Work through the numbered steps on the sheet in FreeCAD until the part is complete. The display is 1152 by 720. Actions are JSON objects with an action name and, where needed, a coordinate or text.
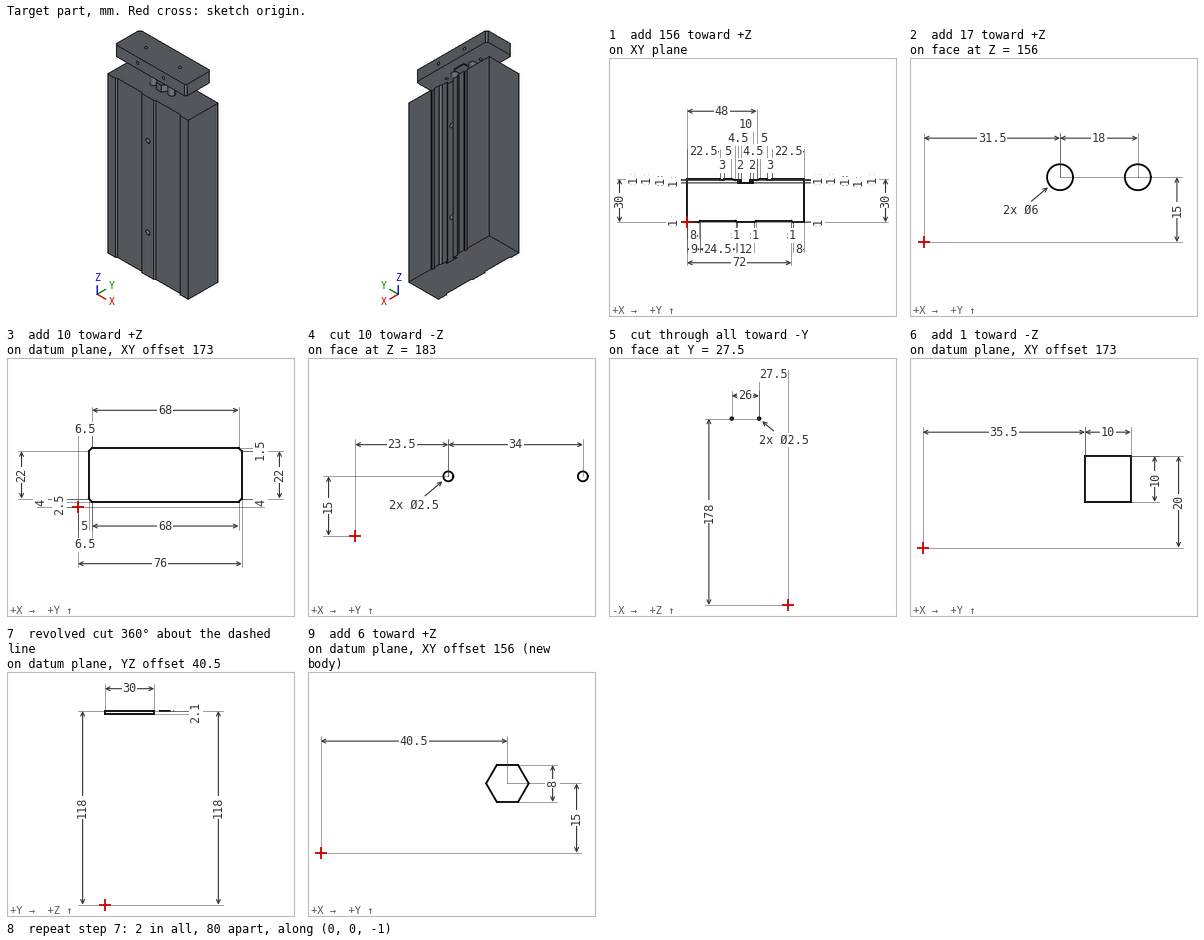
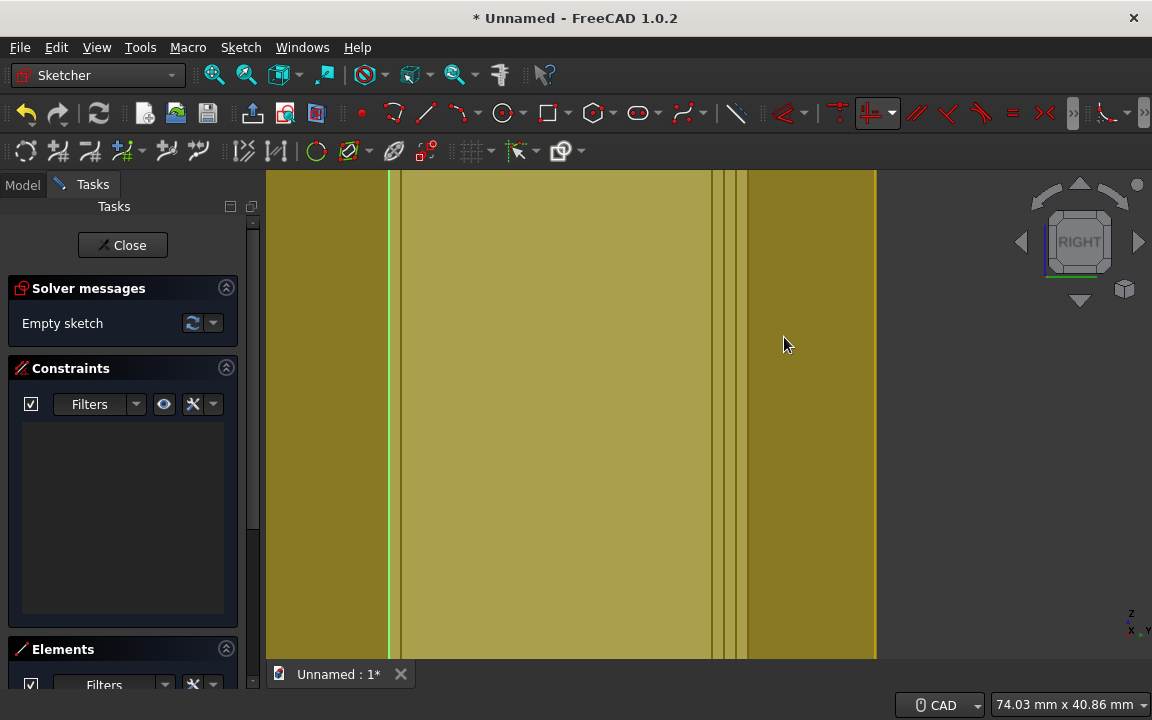
{"action": "key", "text": "g r"}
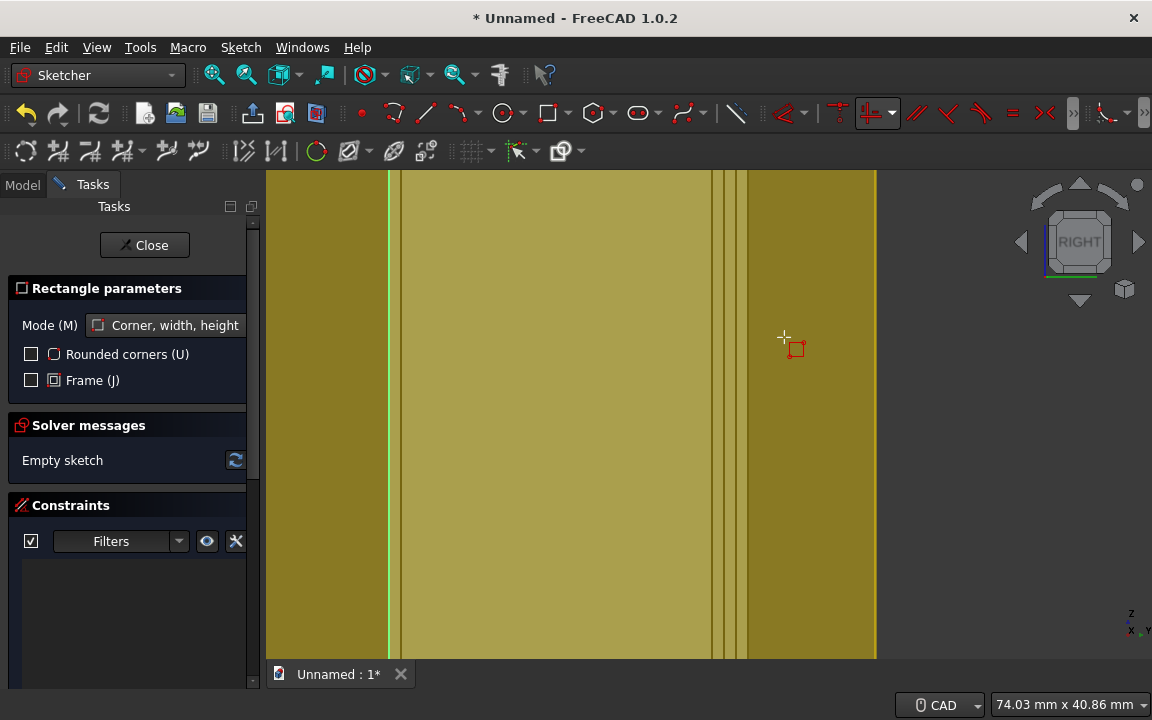
{"action": "left_click", "coordinate": [389, 402]}
{"action": "mouse_move", "coordinate": [748, 427]}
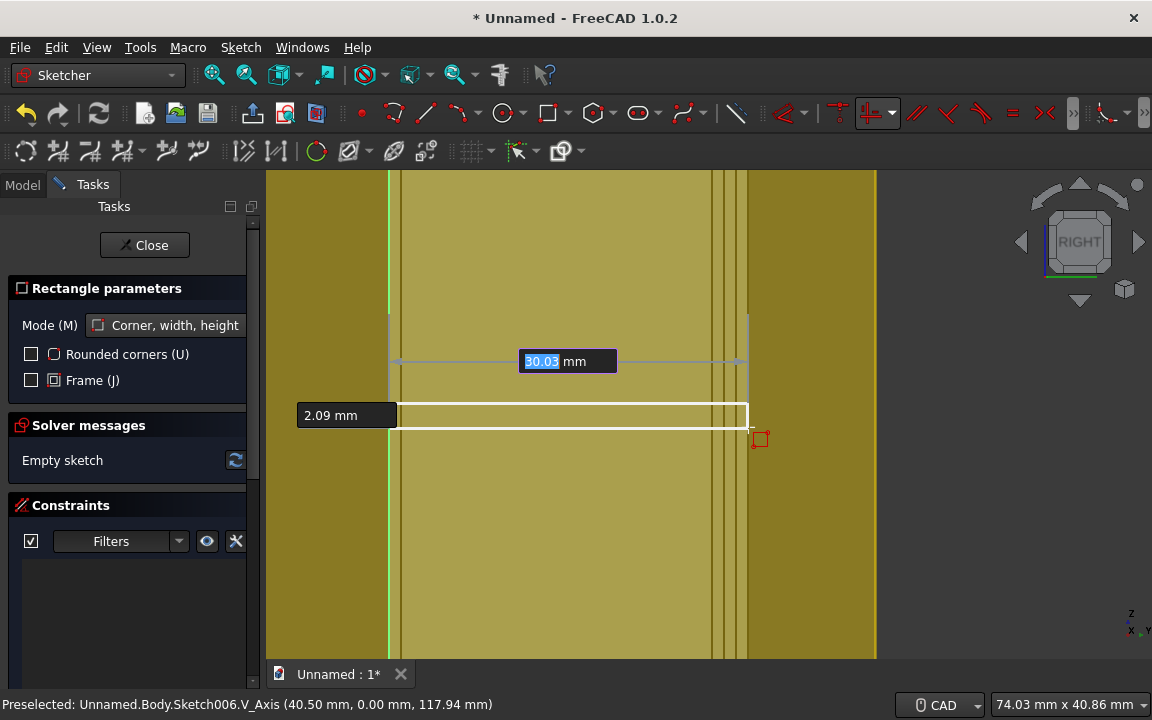
{"action": "type", "text": "30"}
{"action": "key", "text": "Tab"}
{"action": "type", "text": "2.1"}
{"action": "key", "text": "Return"}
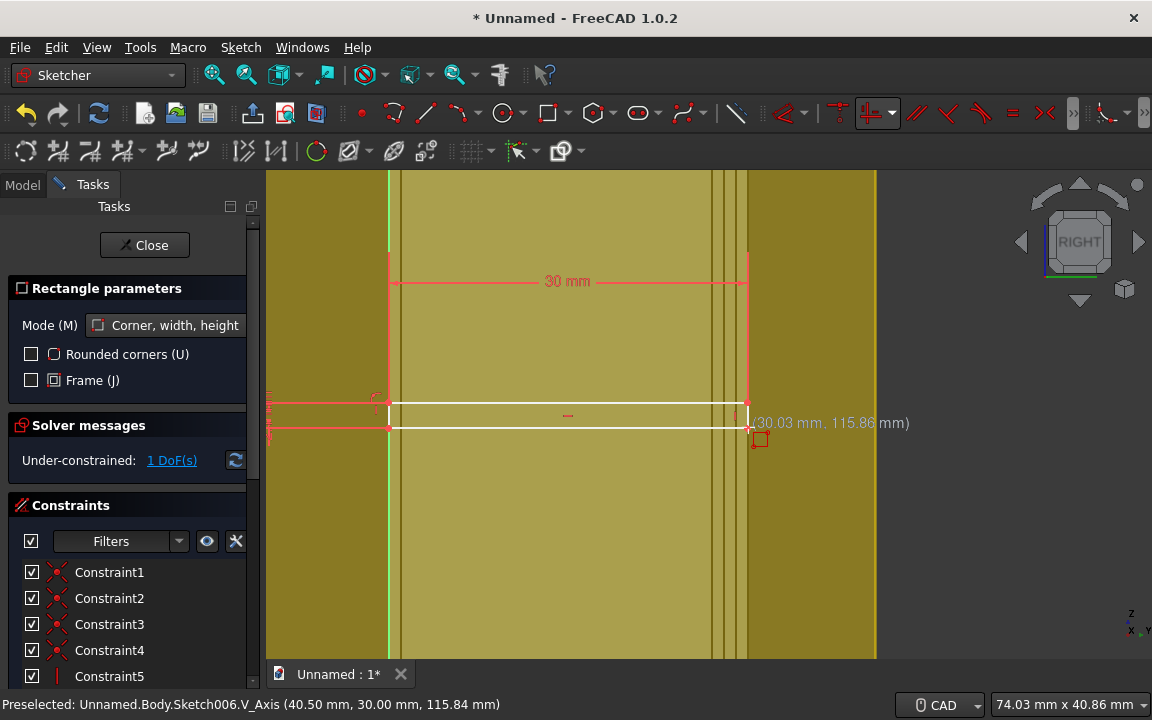
{"action": "key", "text": "g l"}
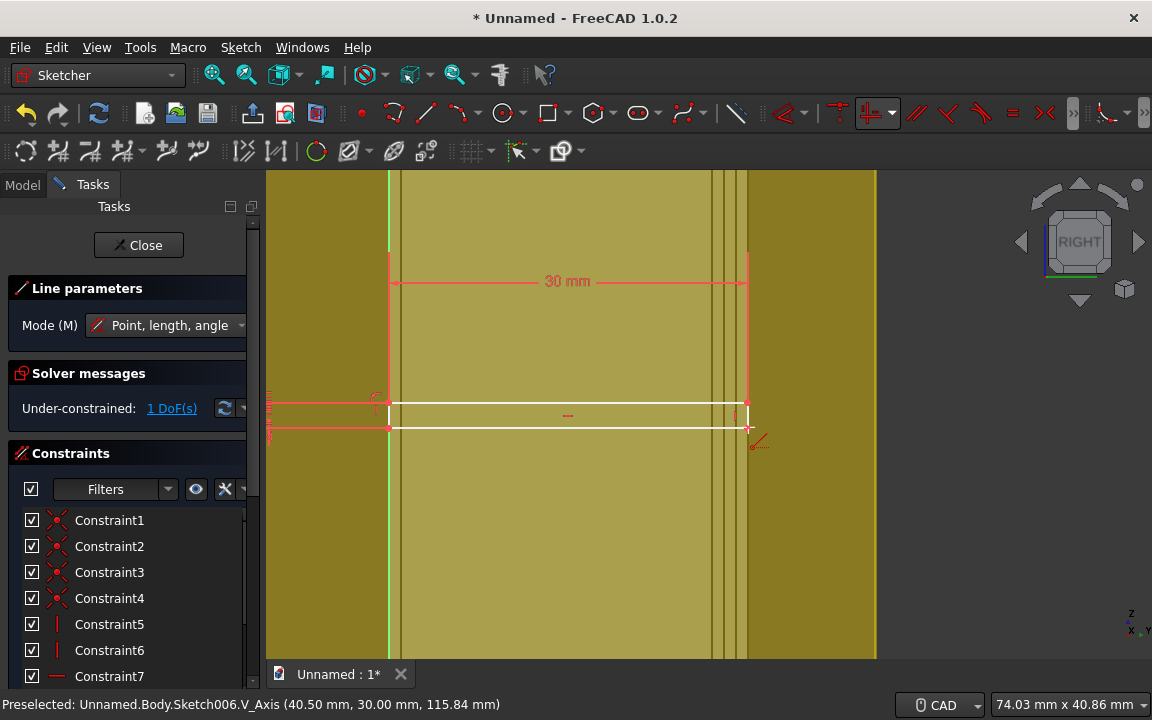
{"action": "left_click", "coordinate": [784, 402]}
{"action": "left_click", "coordinate": [891, 402]}
{"action": "key", "text": "Escape"}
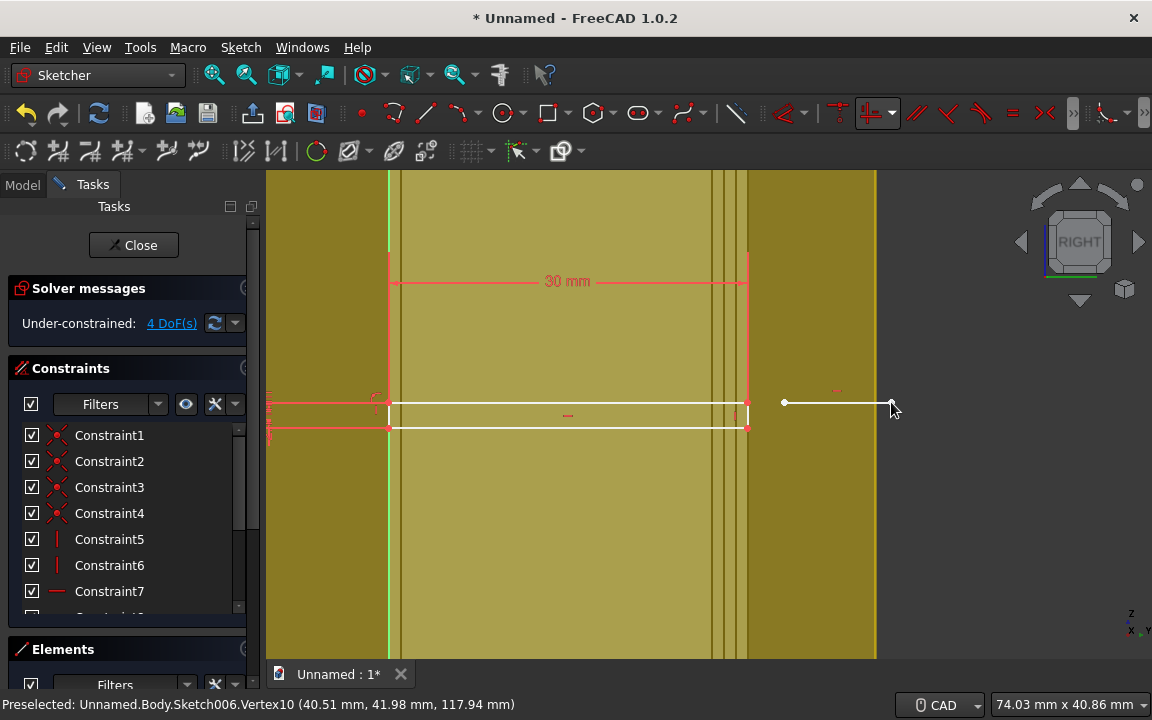
{"action": "left_click", "coordinate": [816, 403]}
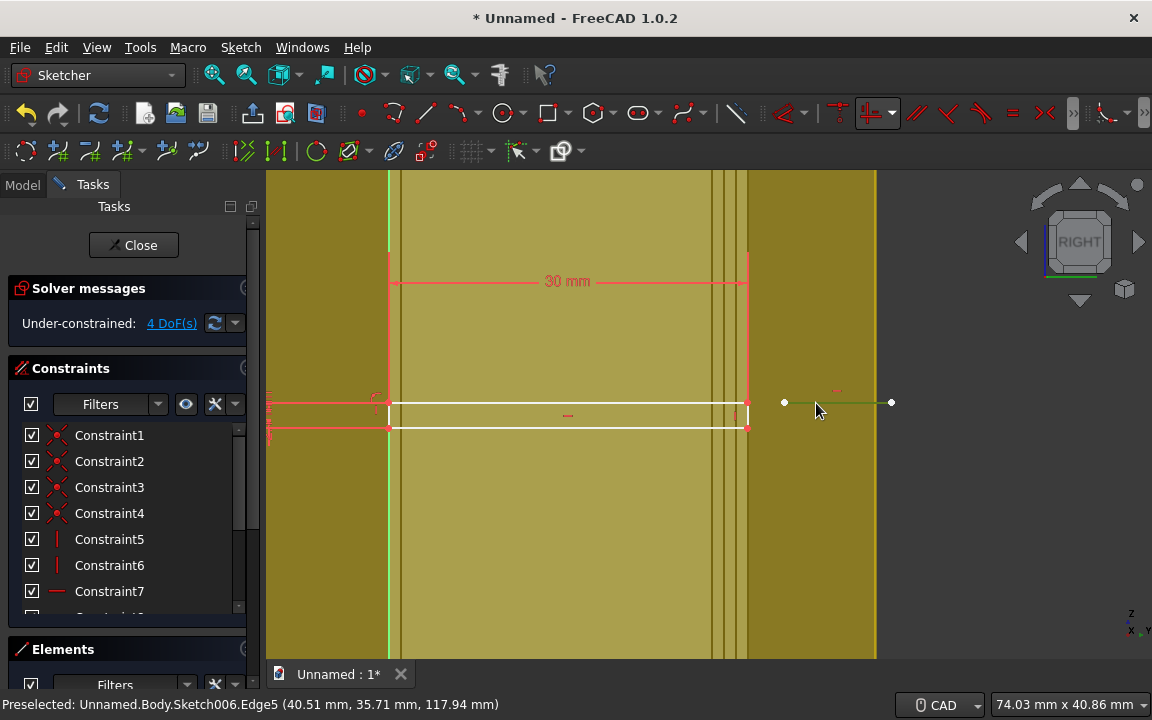
{"action": "left_click", "coordinate": [738, 114]}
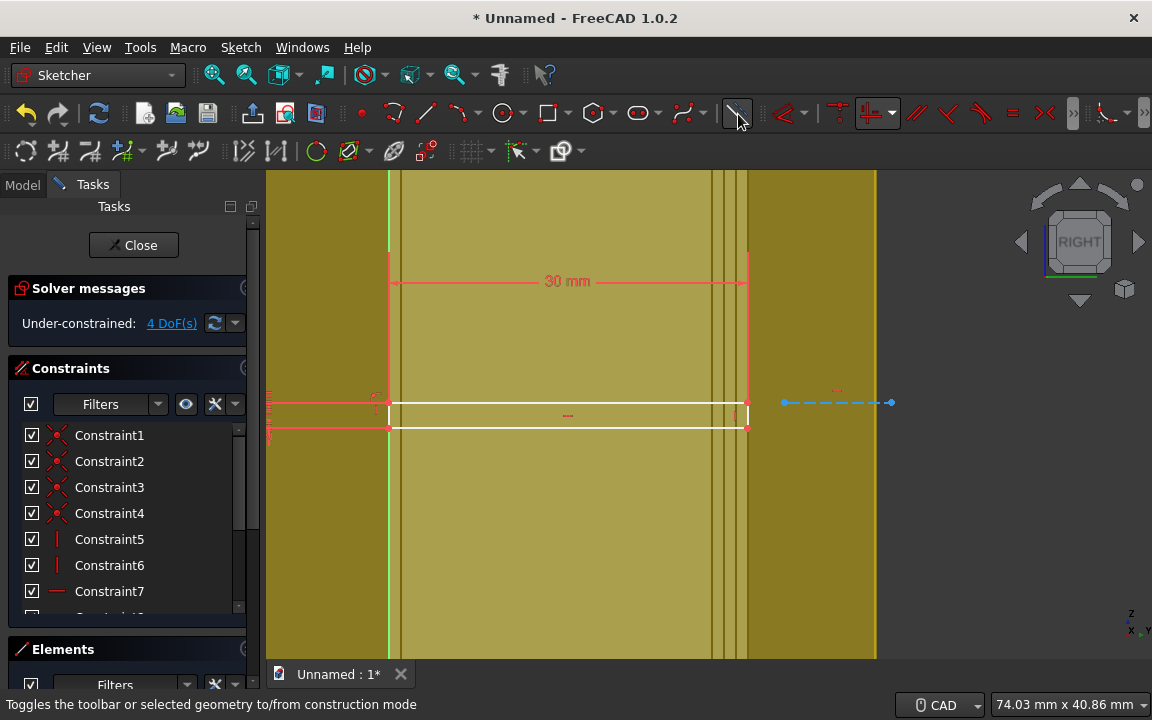
{"action": "left_click", "coordinate": [784, 114]}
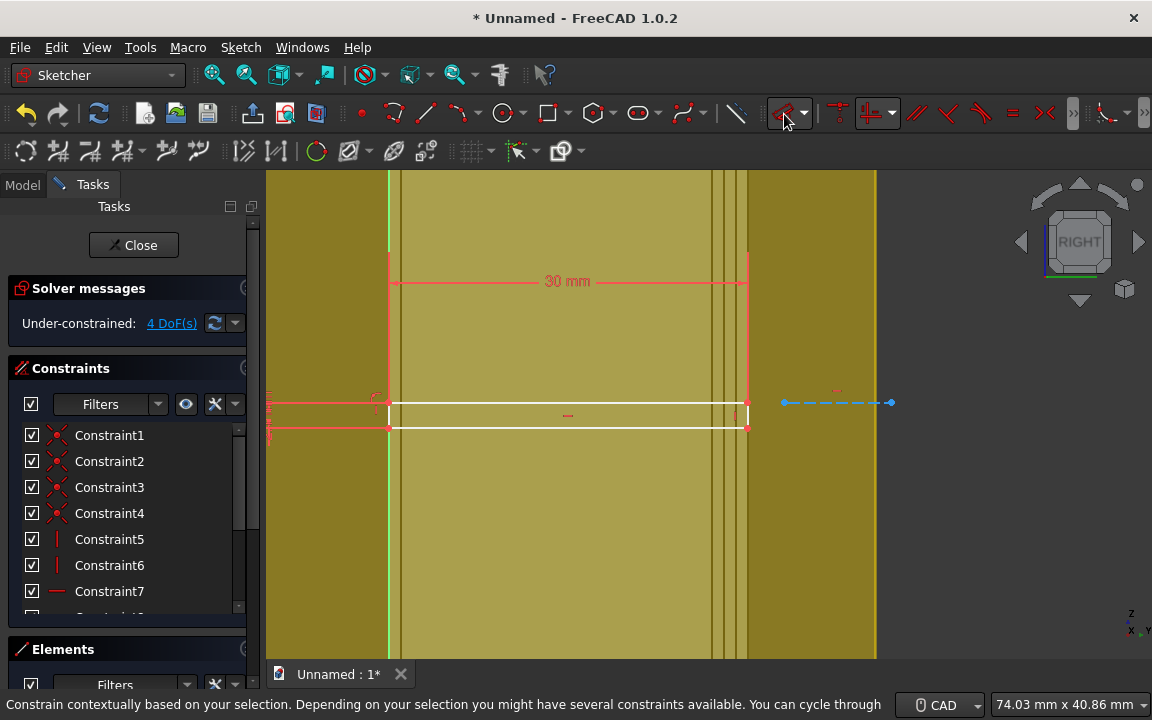
{"action": "left_click", "coordinate": [389, 403]}
{"action": "left_click", "coordinate": [355, 517]}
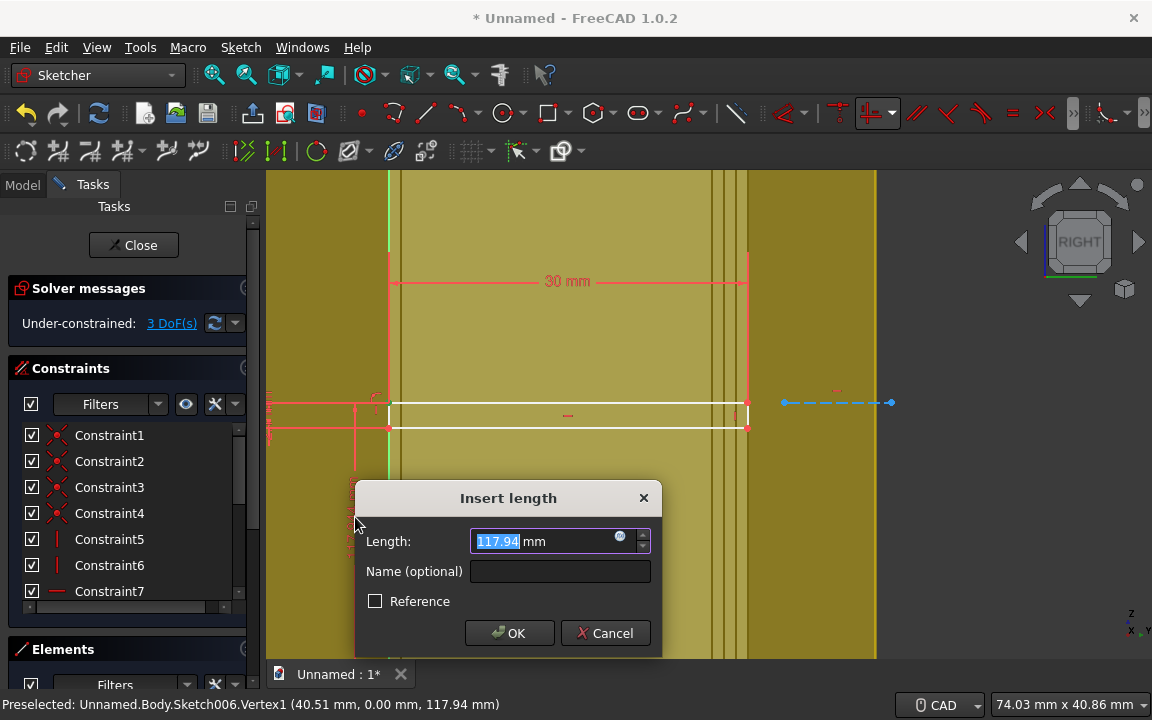
{"action": "type", "text": "118"}
{"action": "key", "text": "Return"}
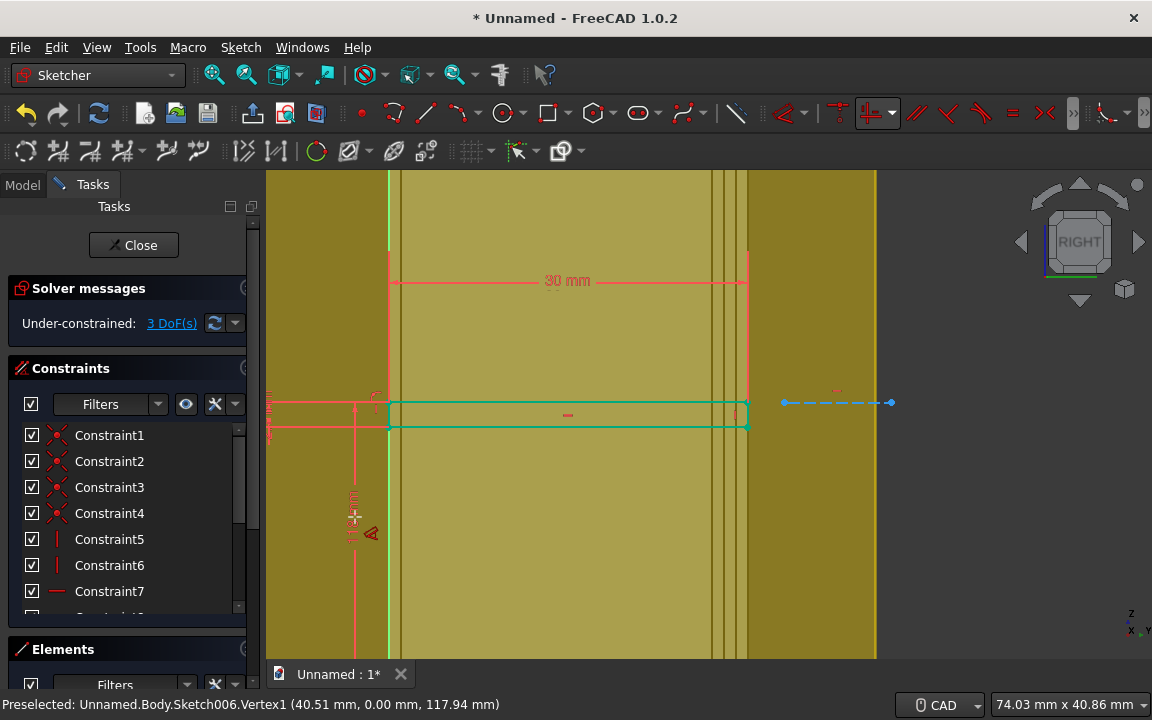
{"action": "left_click", "coordinate": [784, 403]}
{"action": "left_click", "coordinate": [355, 465]}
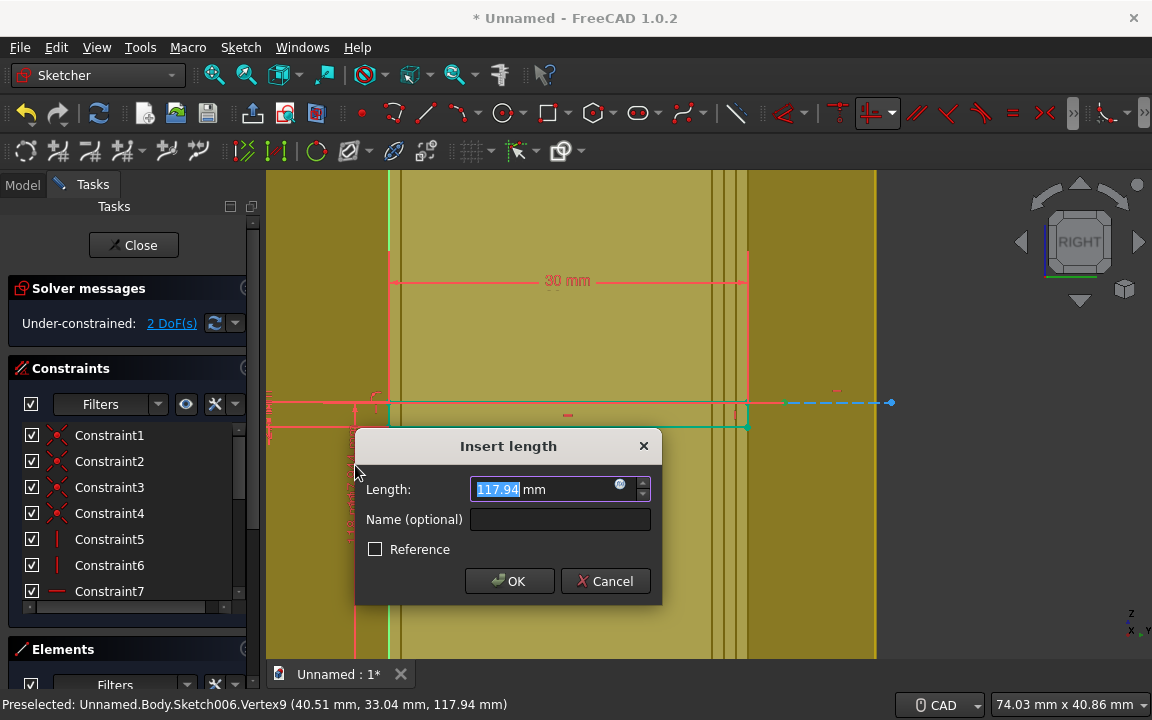
{"action": "type", "text": "118"}
{"action": "key", "text": "Return"}
{"action": "key", "text": "Escape"}